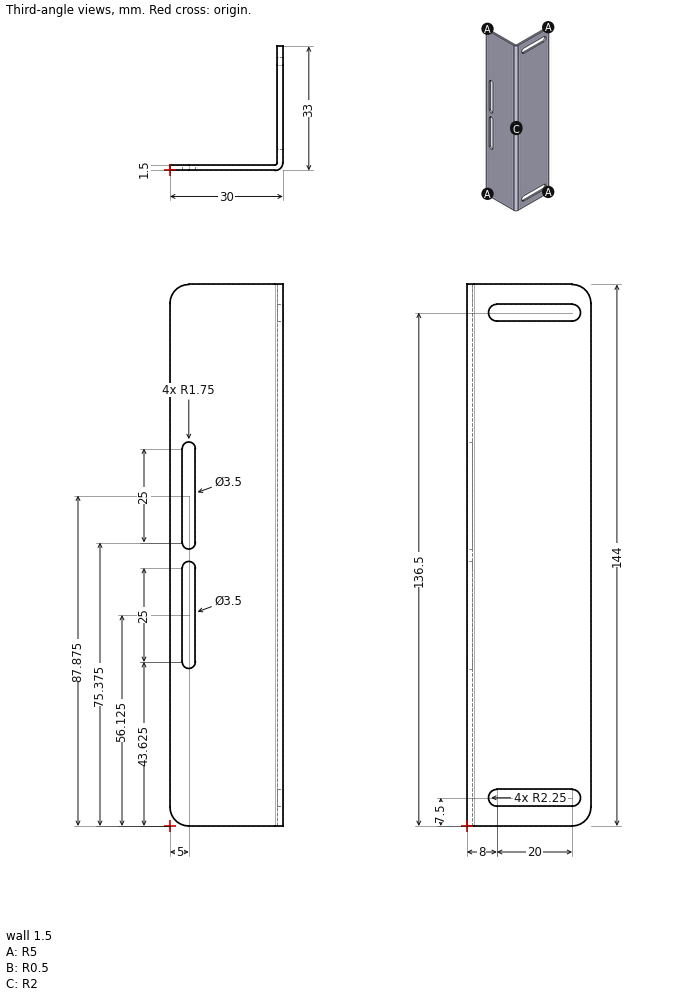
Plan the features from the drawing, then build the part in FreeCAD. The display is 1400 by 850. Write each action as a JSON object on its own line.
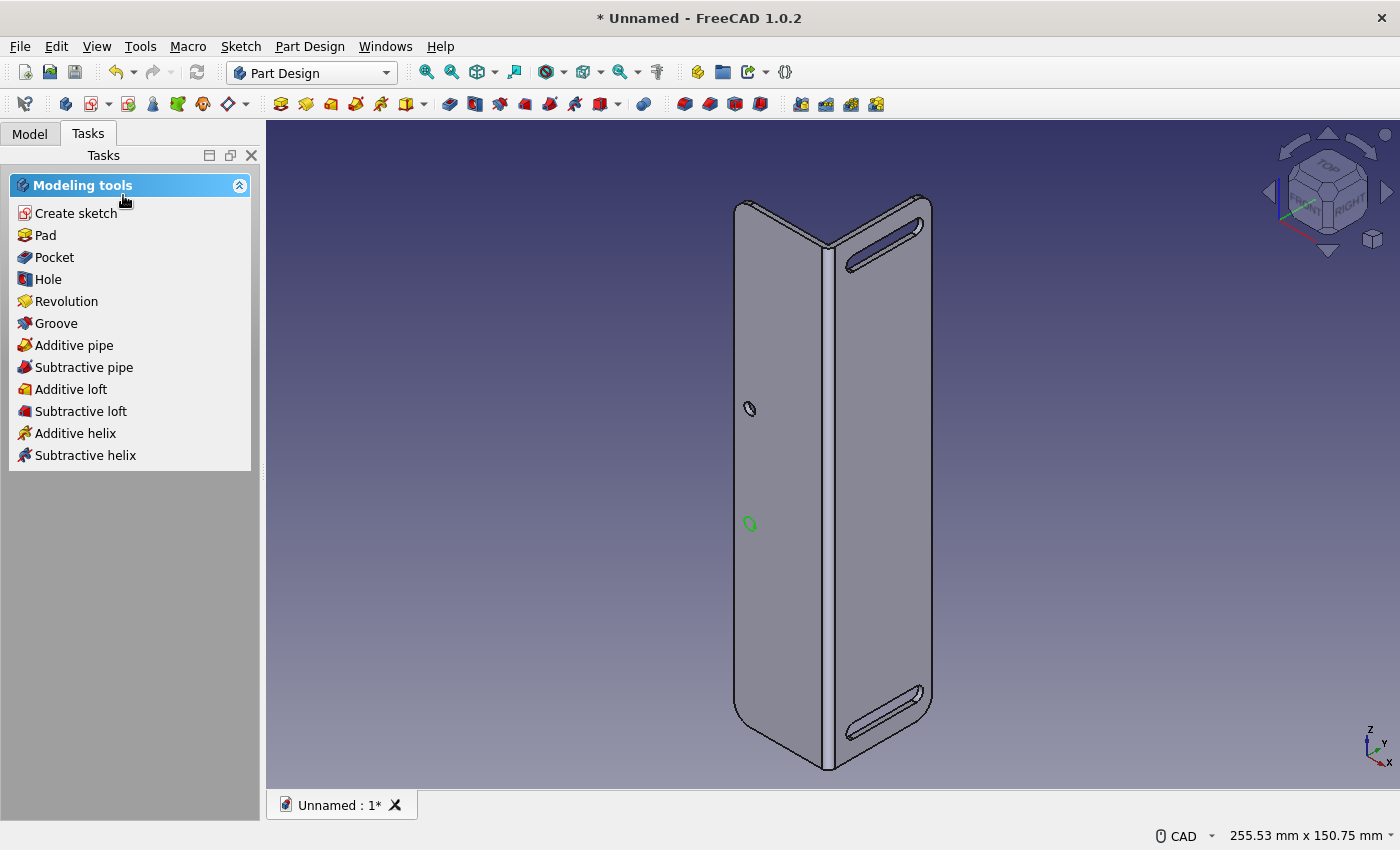
{"action": "left_click", "coordinate": [450, 104]}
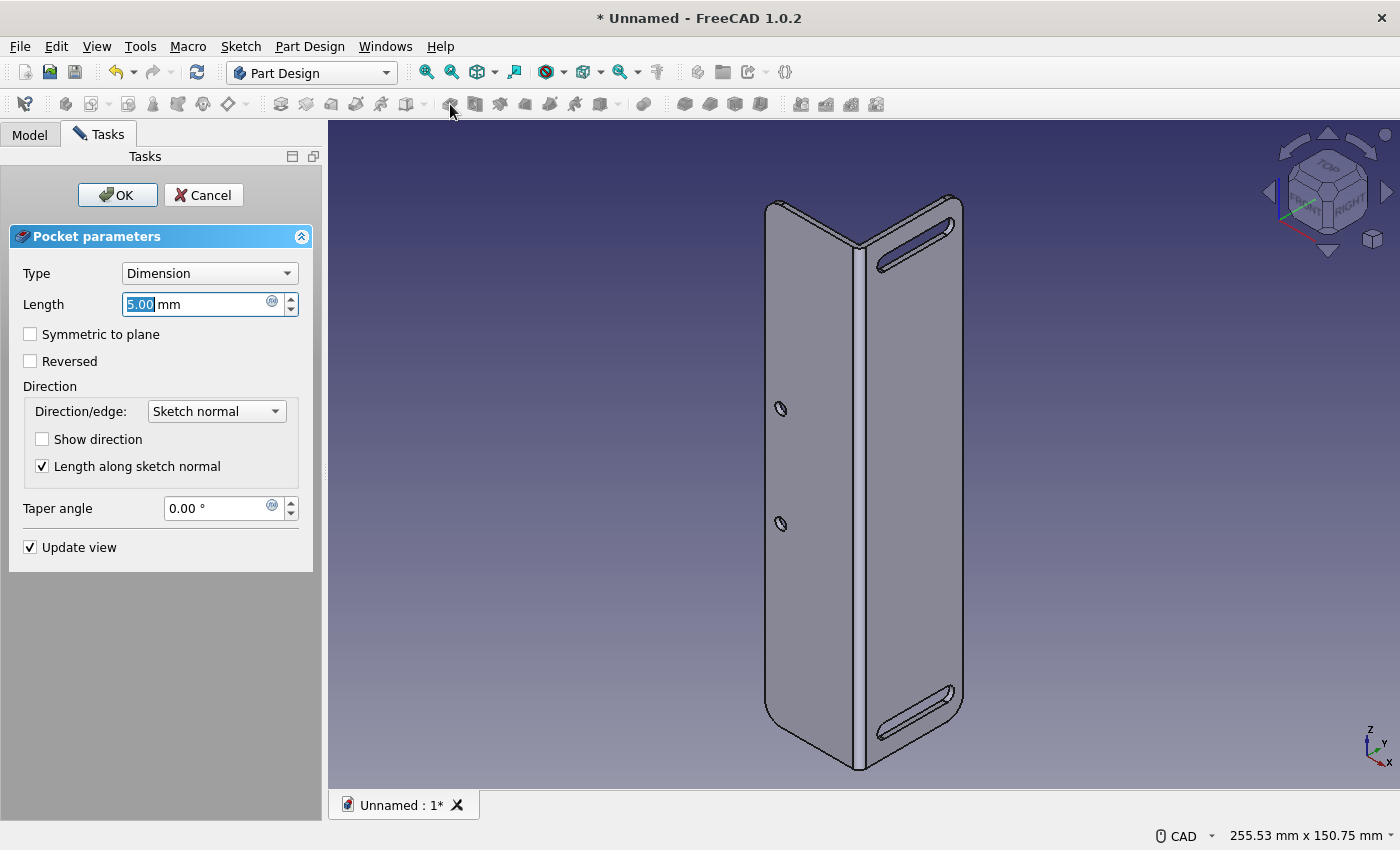
{"action": "left_click", "coordinate": [210, 274]}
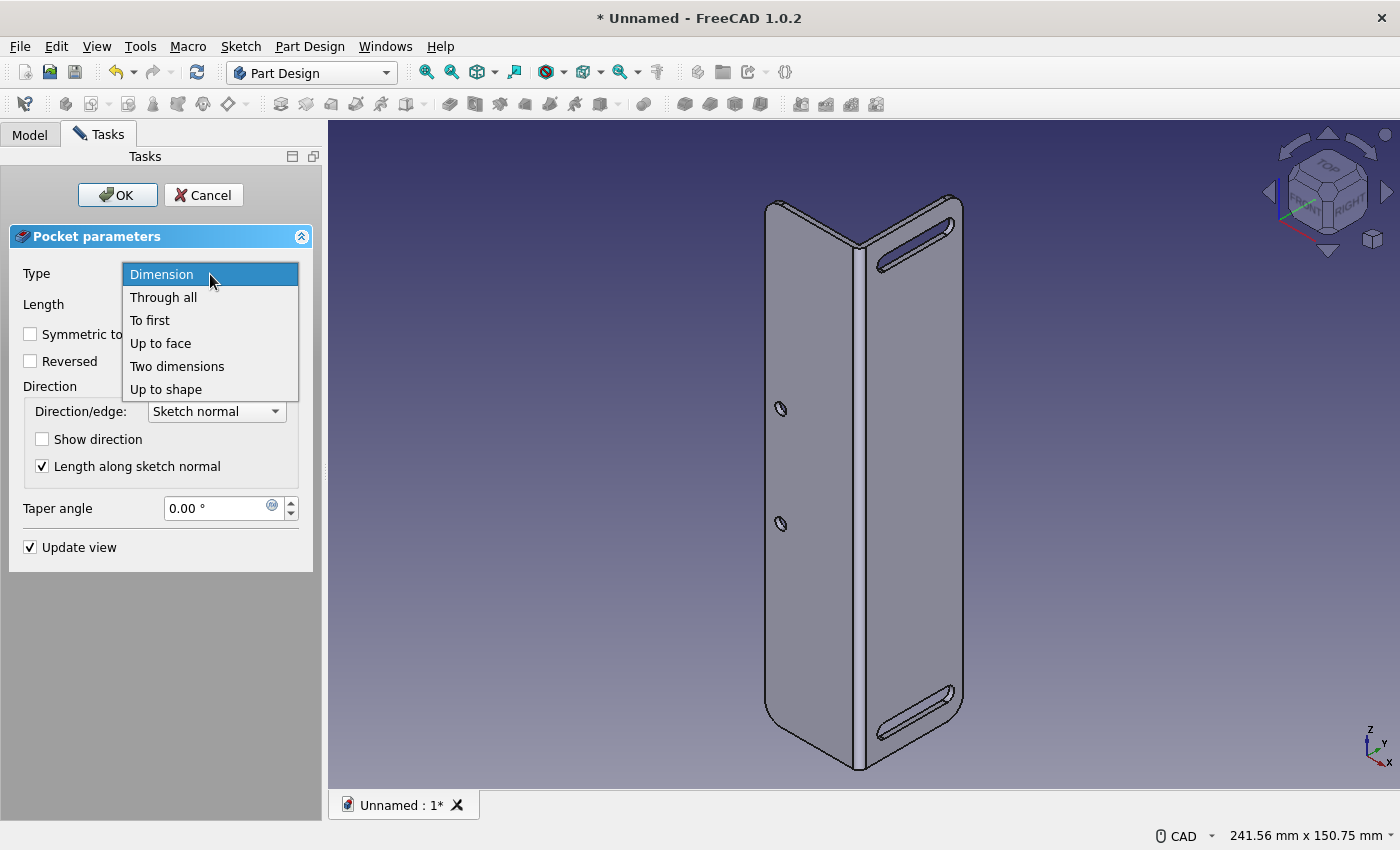
{"action": "left_click", "coordinate": [208, 320]}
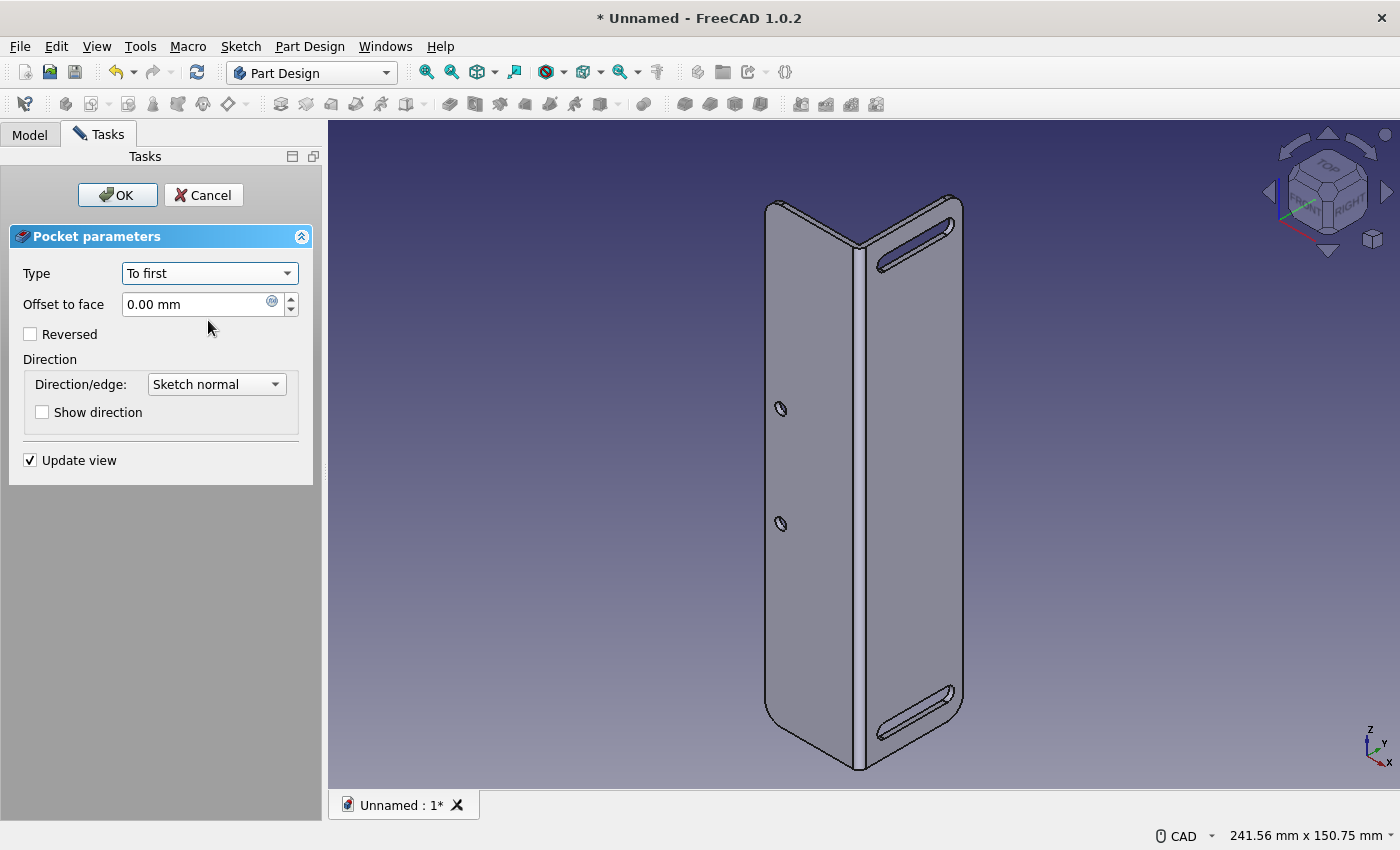
{"action": "left_click", "coordinate": [118, 195]}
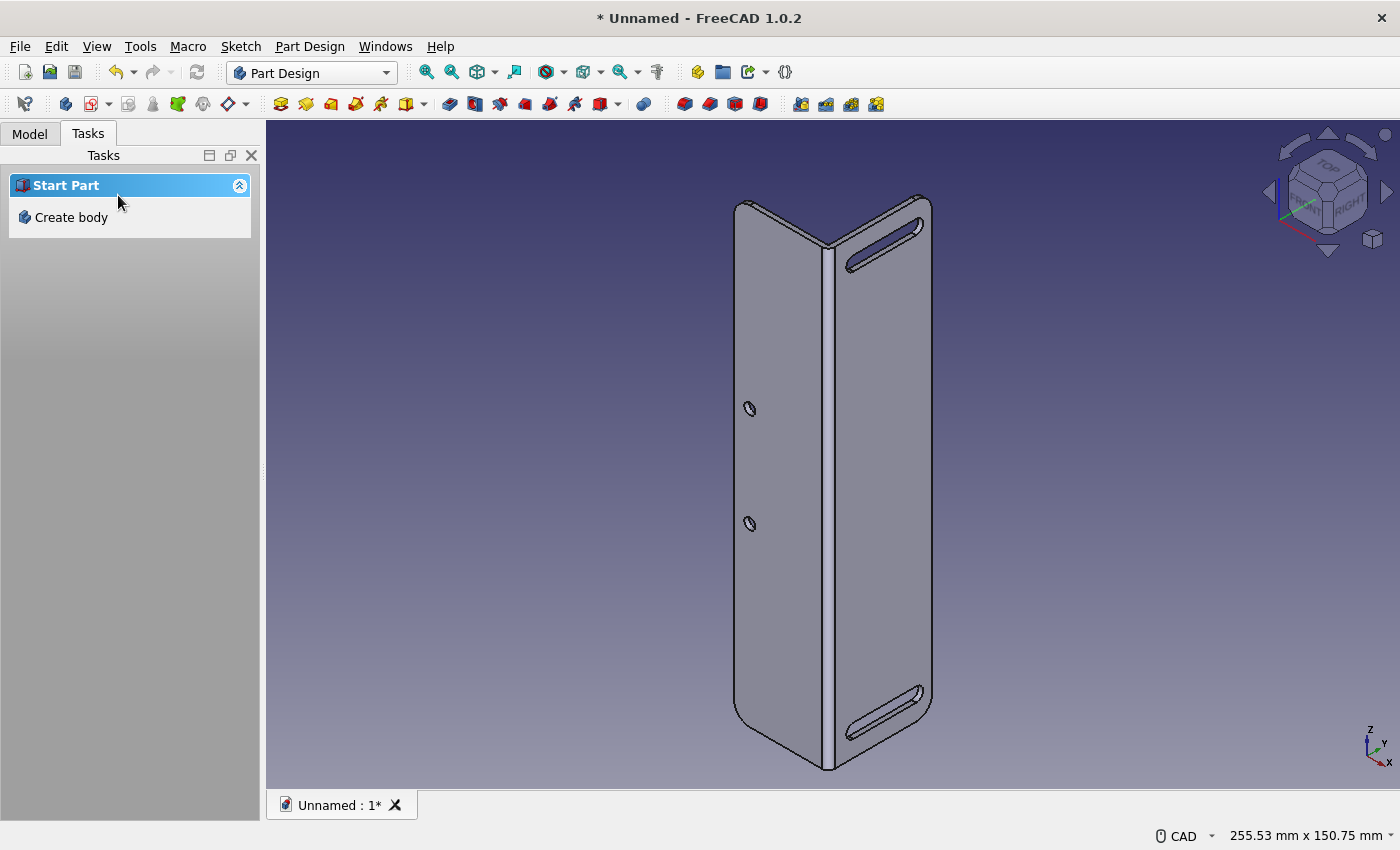
{"action": "left_click", "coordinate": [778, 333]}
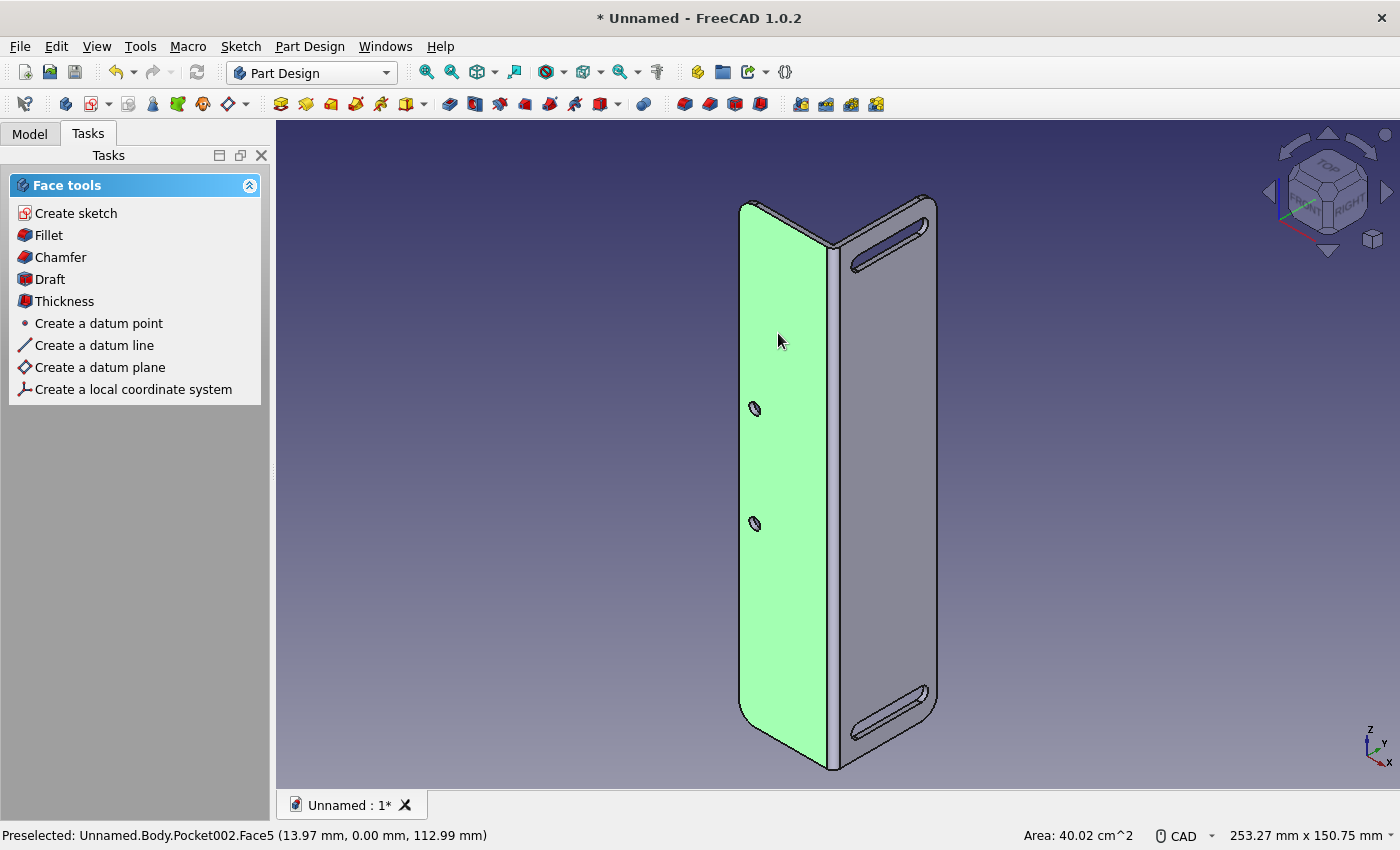
{"action": "left_click", "coordinate": [90, 104]}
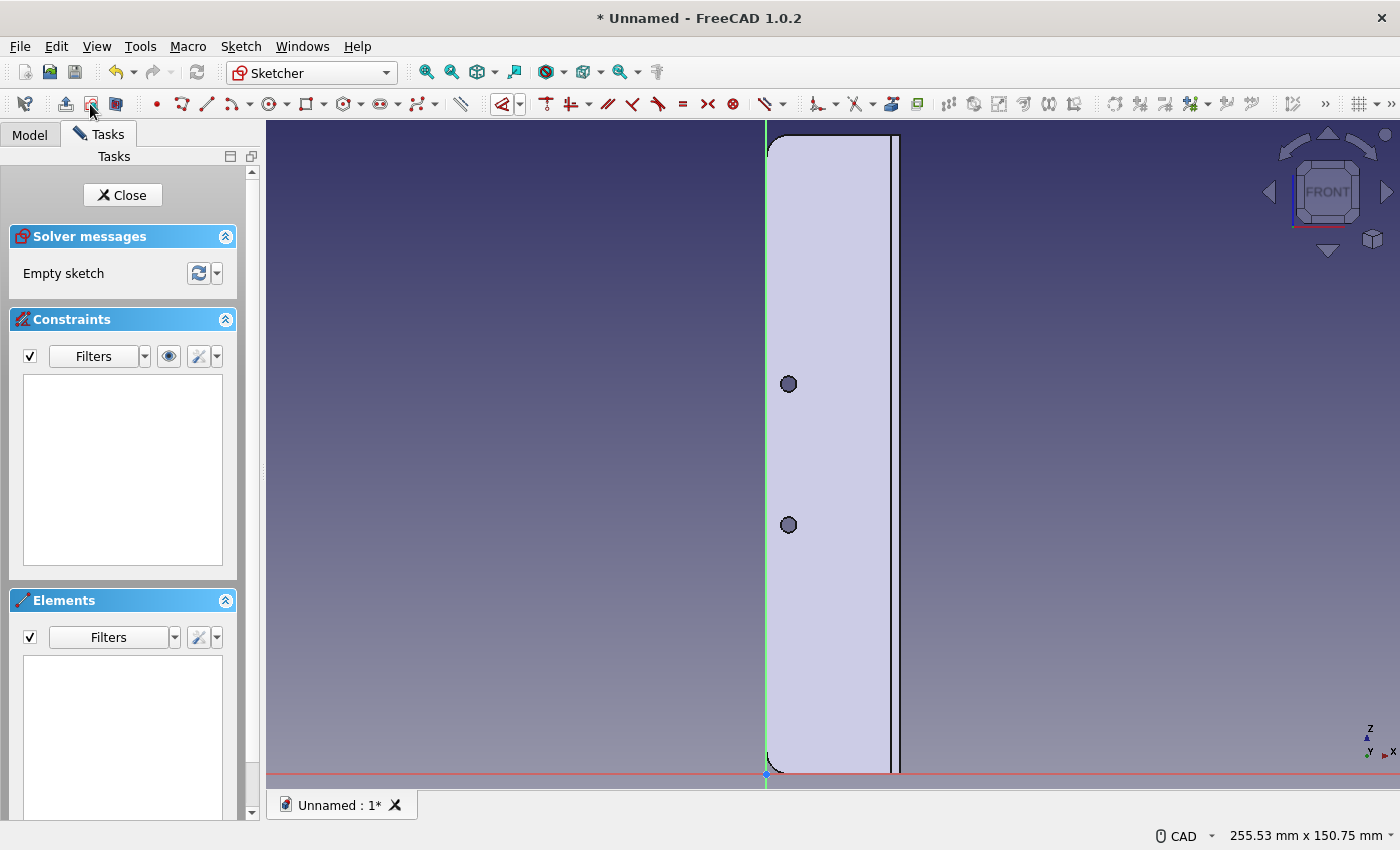
{"action": "scroll", "coordinate": [688, 148], "scroll_direction": "down", "scroll_amount": 1}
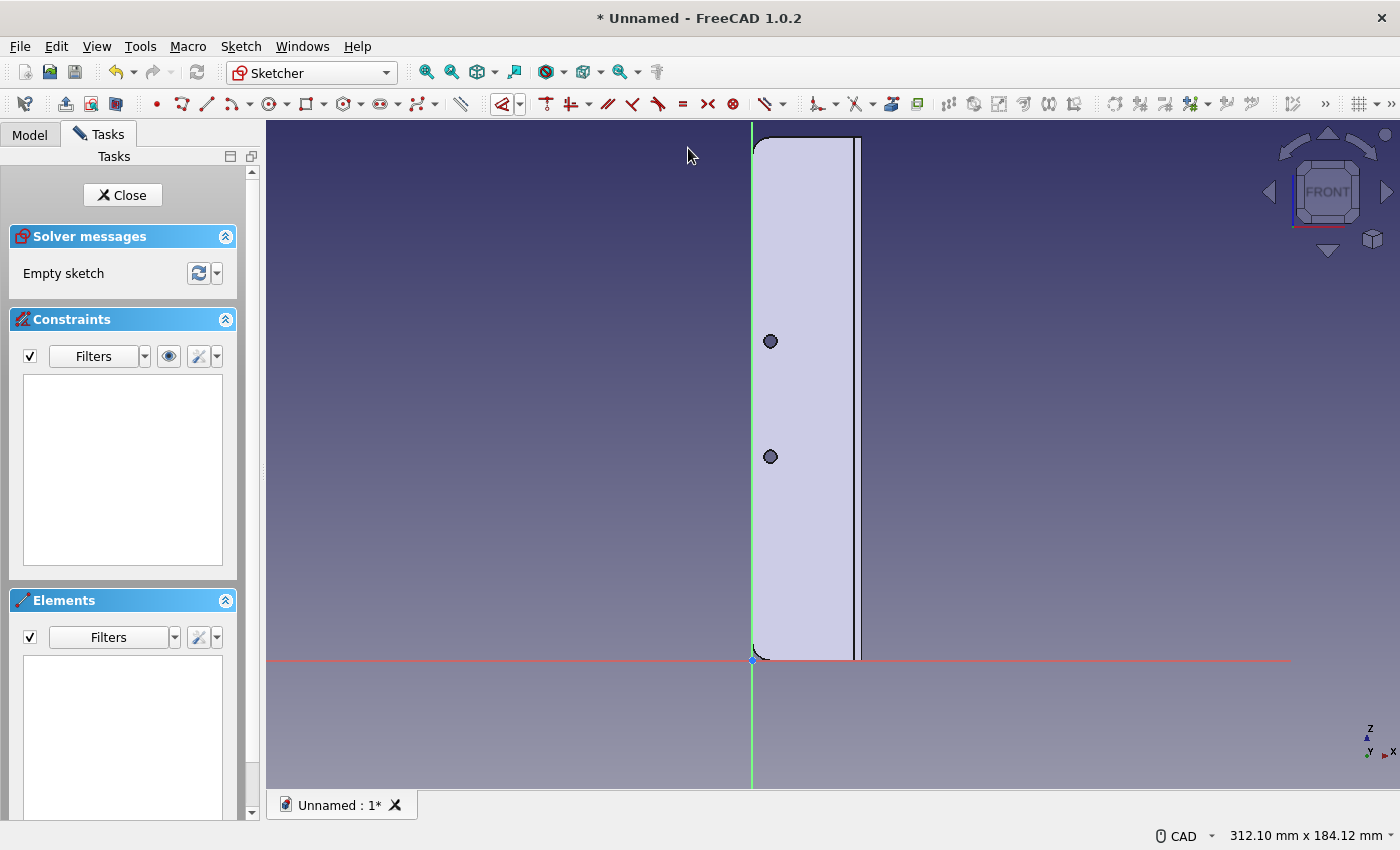
{"action": "left_click", "coordinate": [380, 104]}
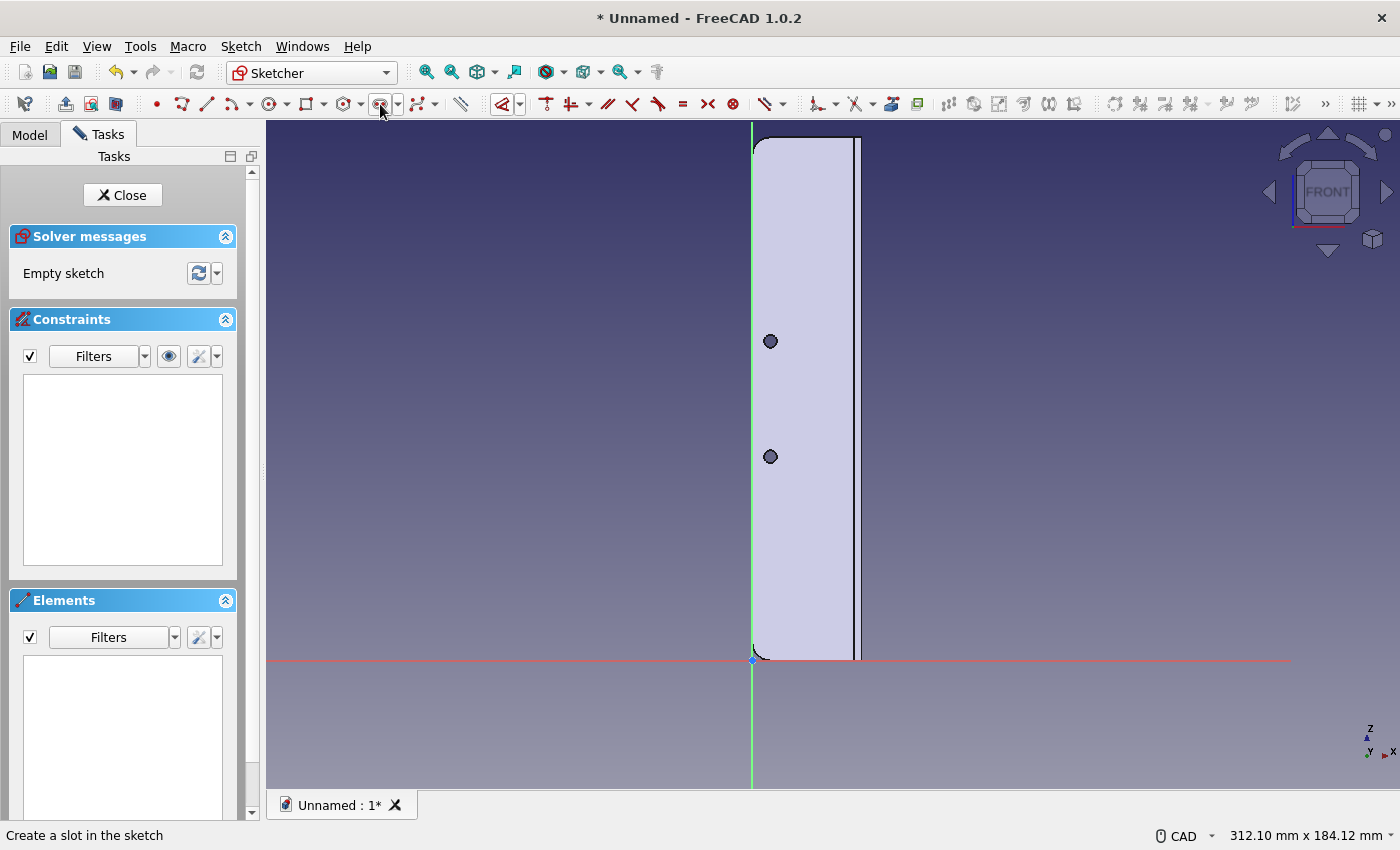
{"action": "scroll", "coordinate": [770, 387], "scroll_direction": "up", "scroll_amount": 7}